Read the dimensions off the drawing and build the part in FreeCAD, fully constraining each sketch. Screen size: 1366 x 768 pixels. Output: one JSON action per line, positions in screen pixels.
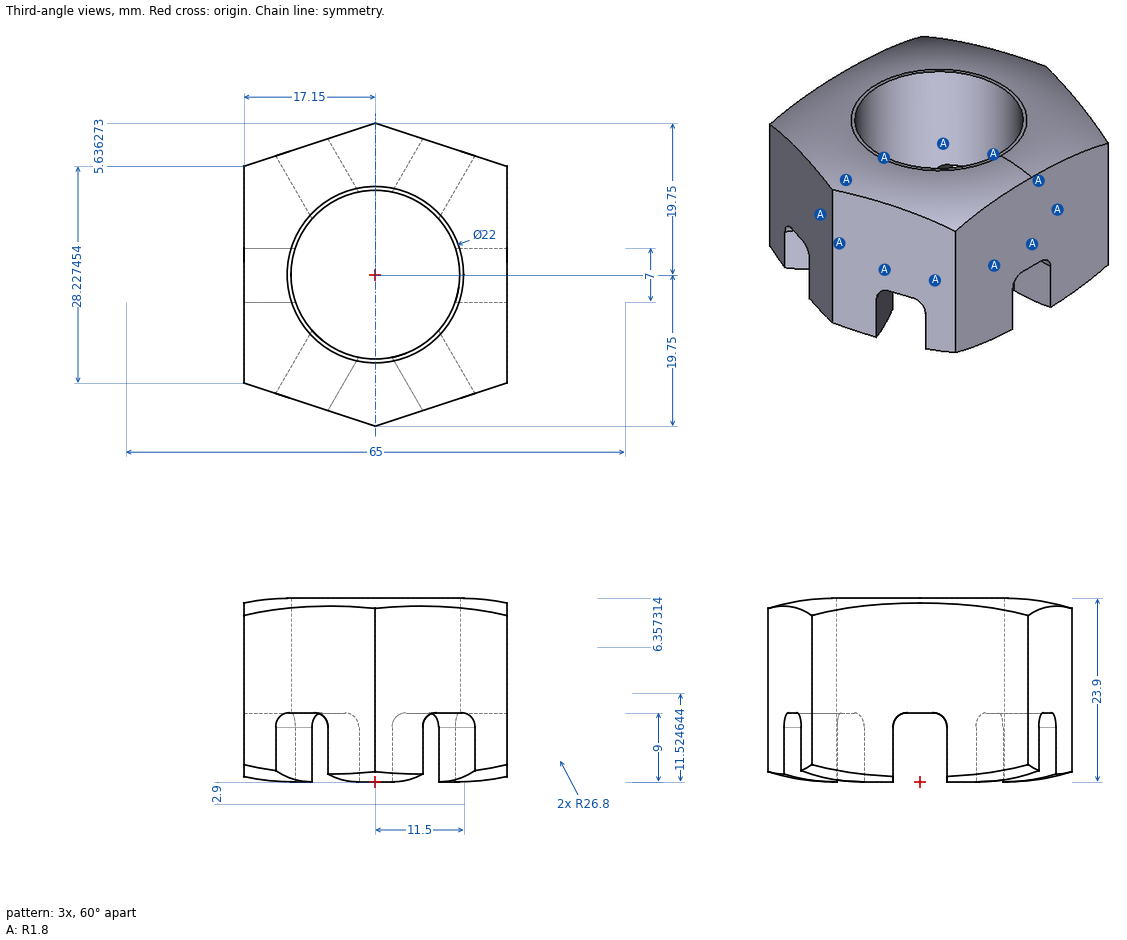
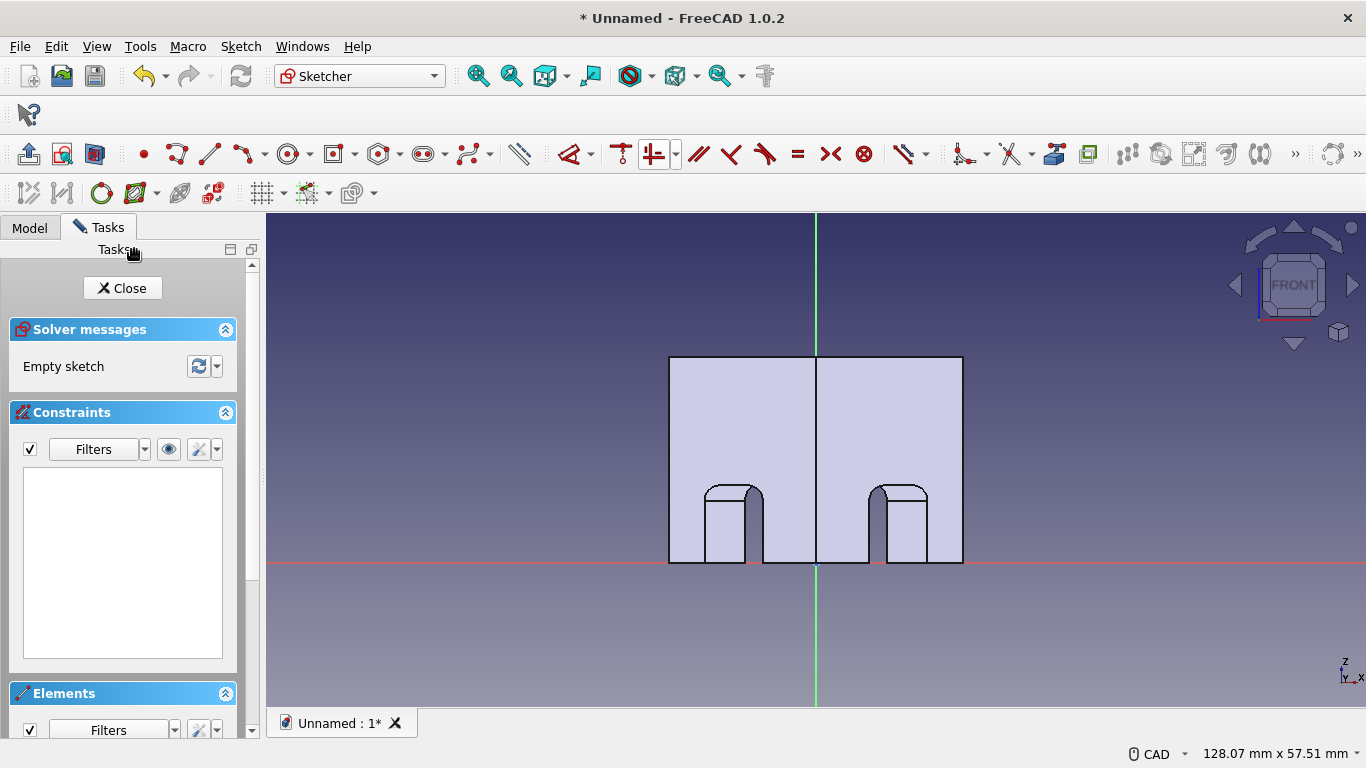
{"action": "left_click", "coordinate": [95, 154]}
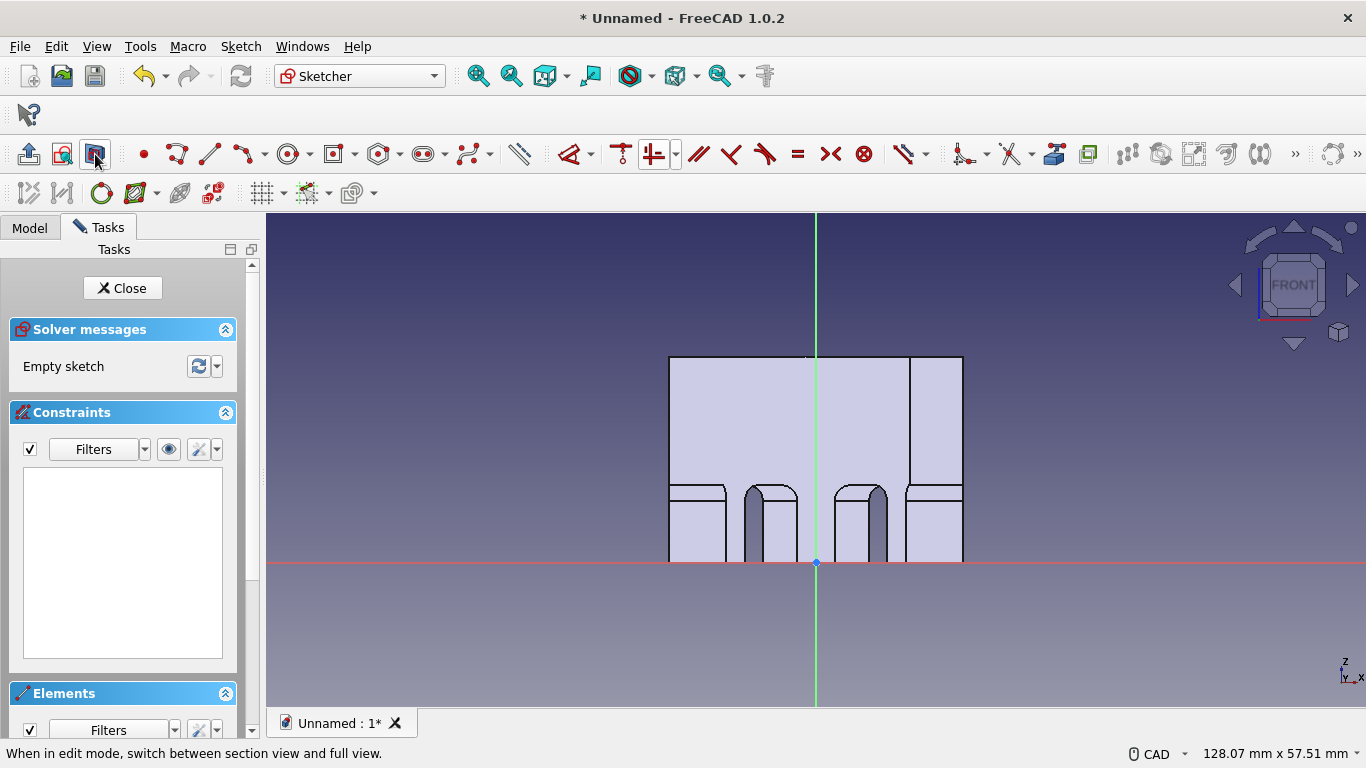
{"action": "scroll", "coordinate": [1201, 460], "scroll_direction": "up", "scroll_amount": 2}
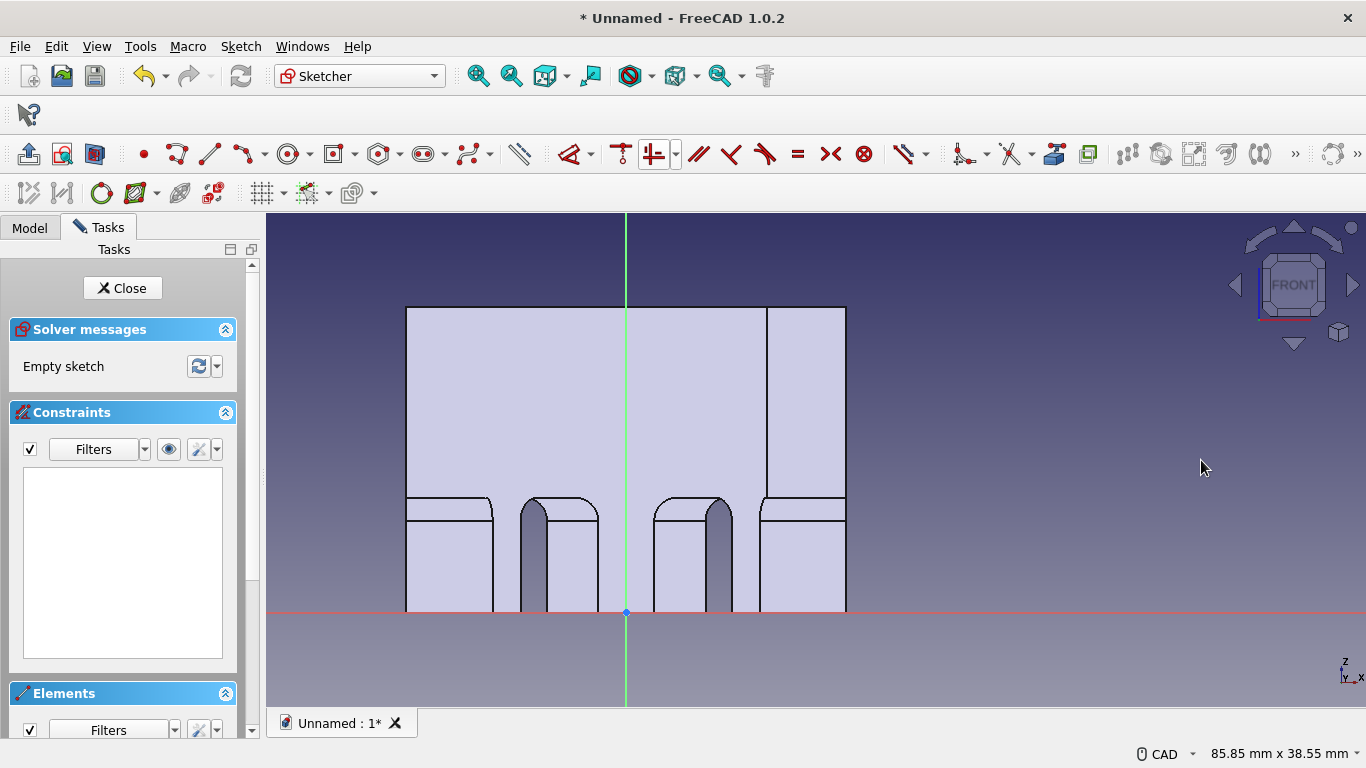
{"action": "left_click", "coordinate": [177, 154]}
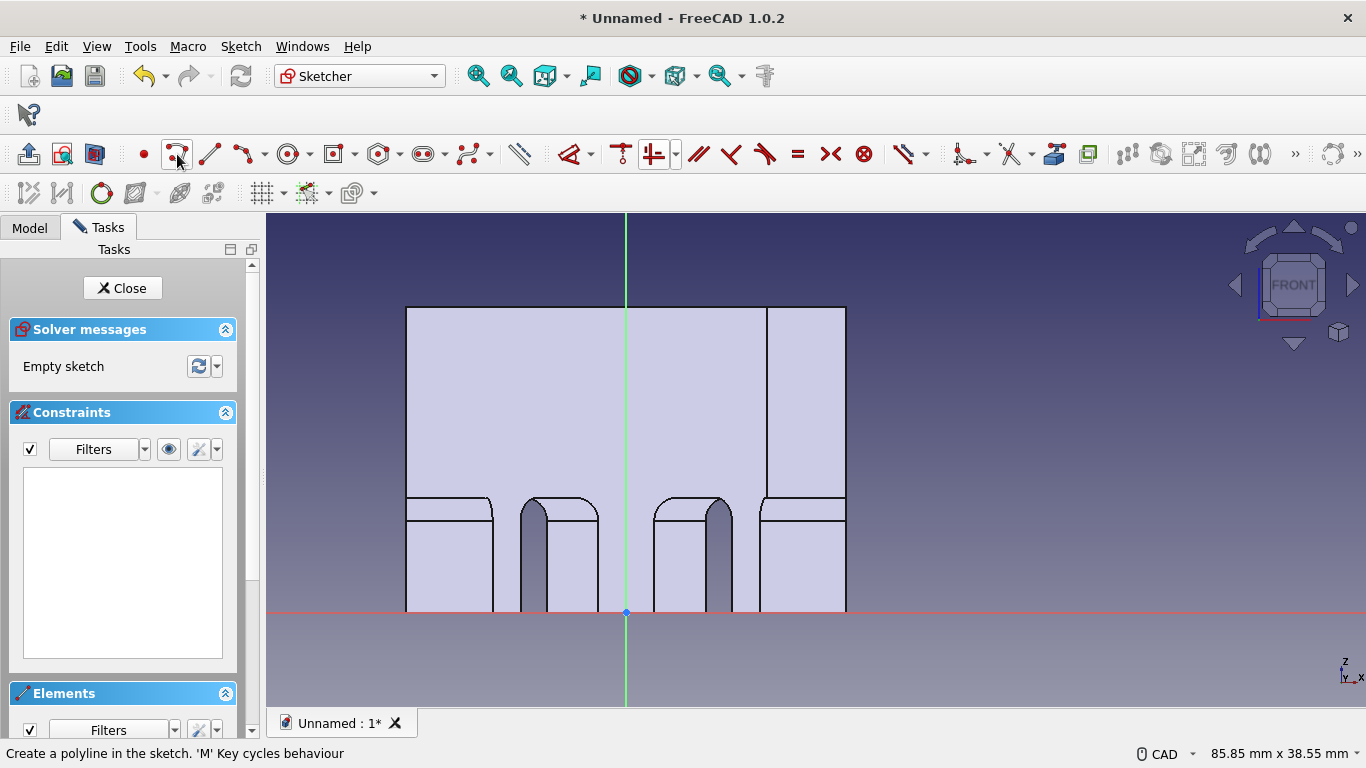
{"action": "left_click", "coordinate": [1056, 465]}
{"action": "left_click", "coordinate": [1056, 613]}
{"action": "left_click", "coordinate": [774, 604]}
{"action": "right_click", "coordinate": [774, 604]}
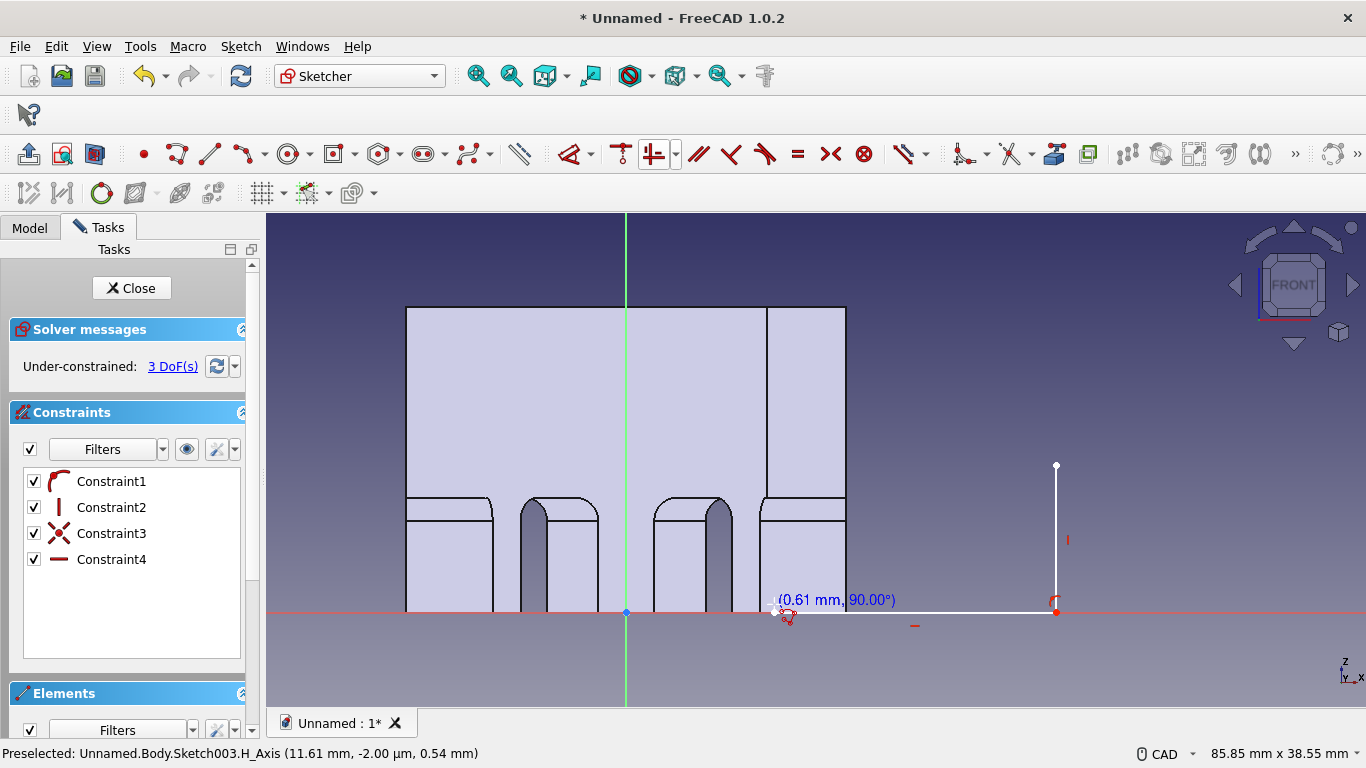
{"action": "left_click", "coordinate": [242, 154]}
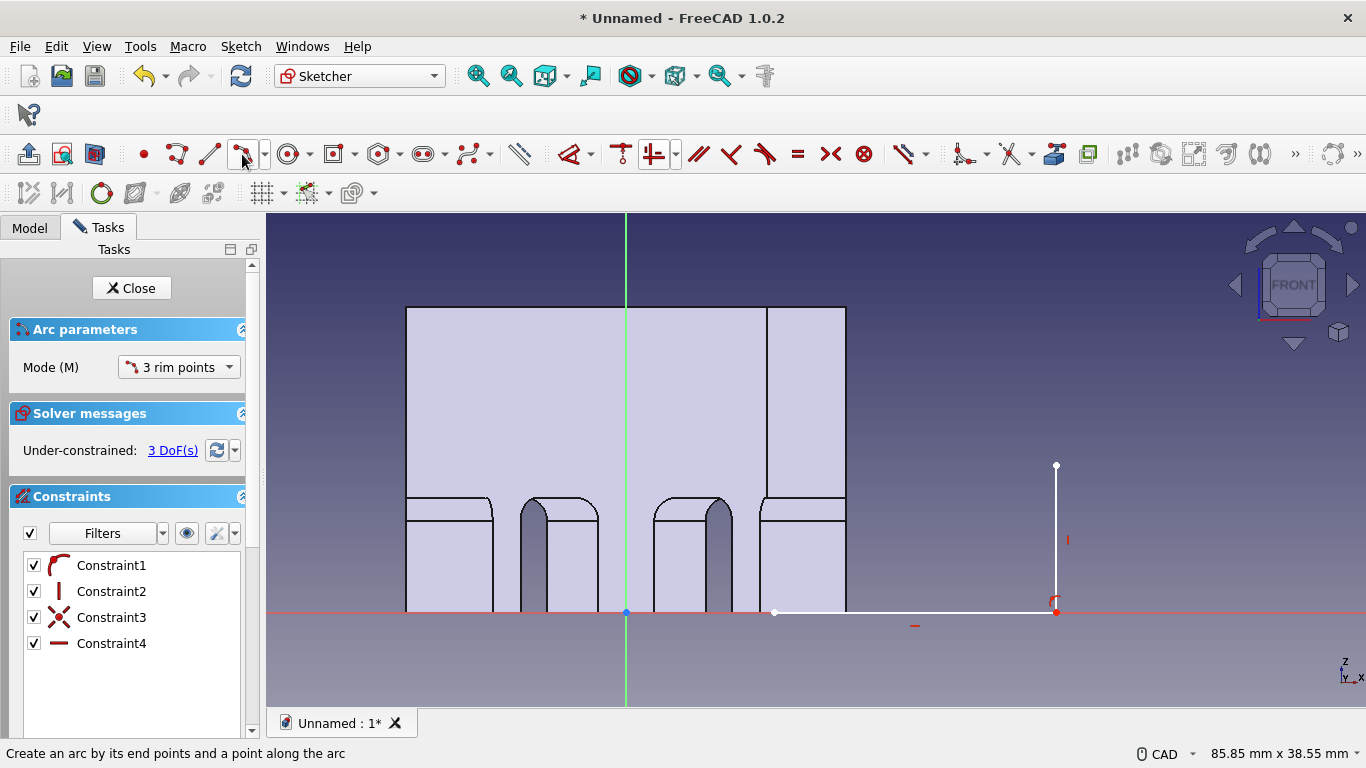
{"action": "left_click", "coordinate": [774, 613]}
{"action": "left_click", "coordinate": [1056, 466]}
{"action": "left_click", "coordinate": [933, 574]}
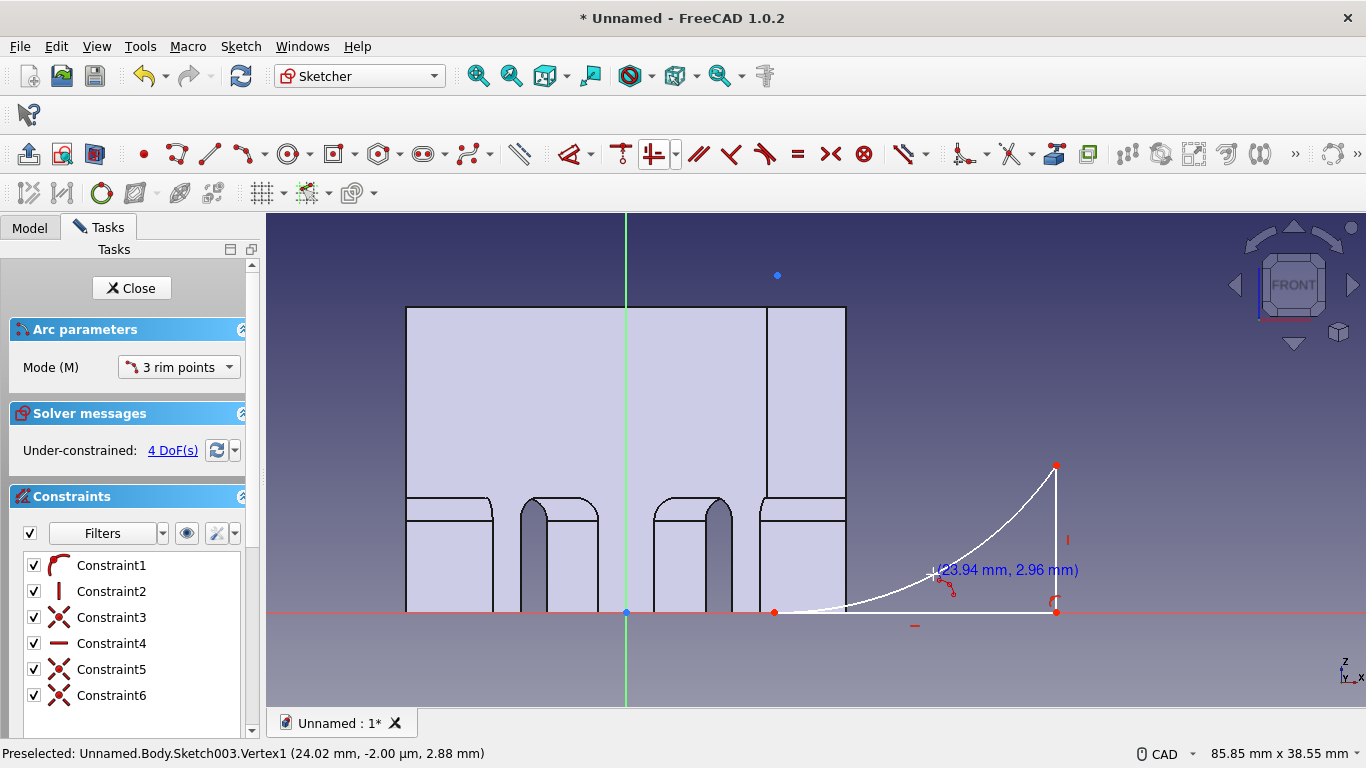
{"action": "left_click", "coordinate": [177, 154]}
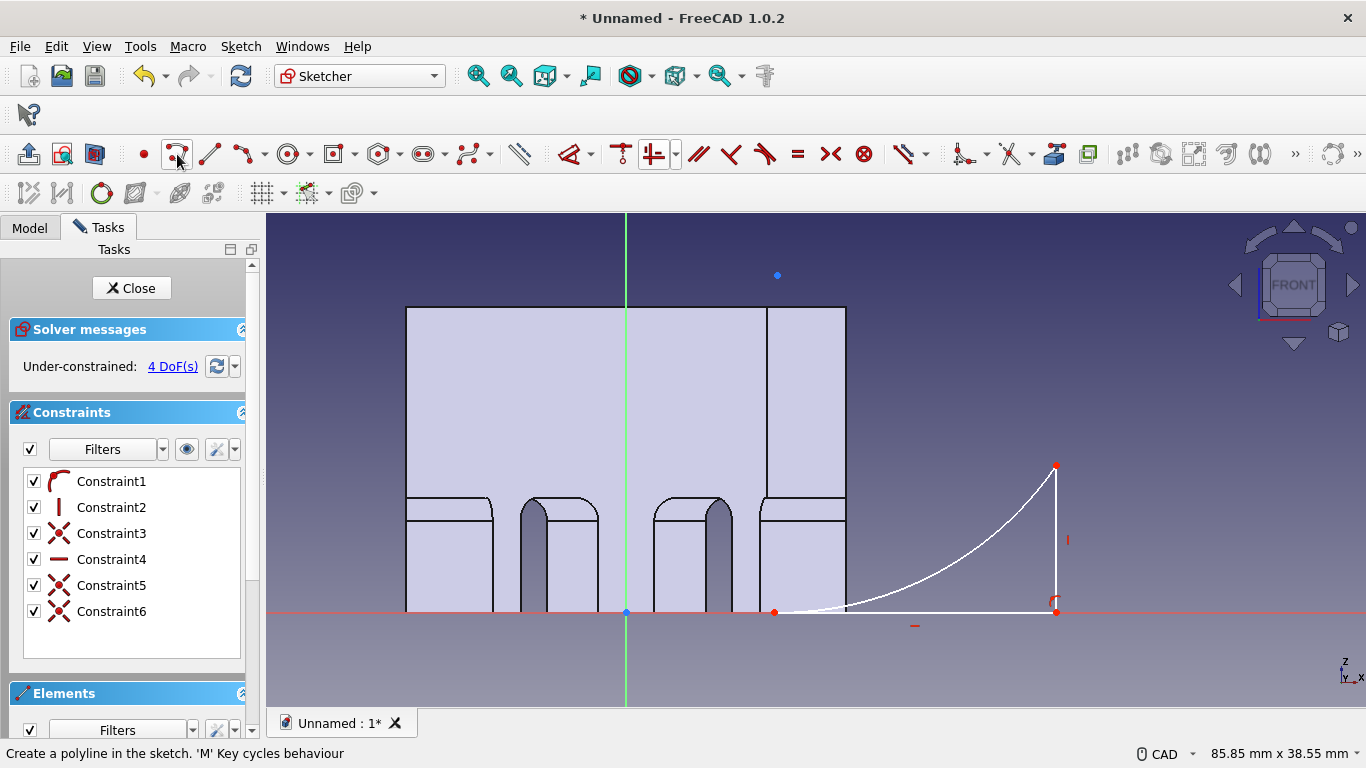
{"action": "left_click", "coordinate": [774, 307]}
{"action": "left_click", "coordinate": [996, 307]}
{"action": "left_click", "coordinate": [996, 388]}
{"action": "right_click", "coordinate": [996, 388]}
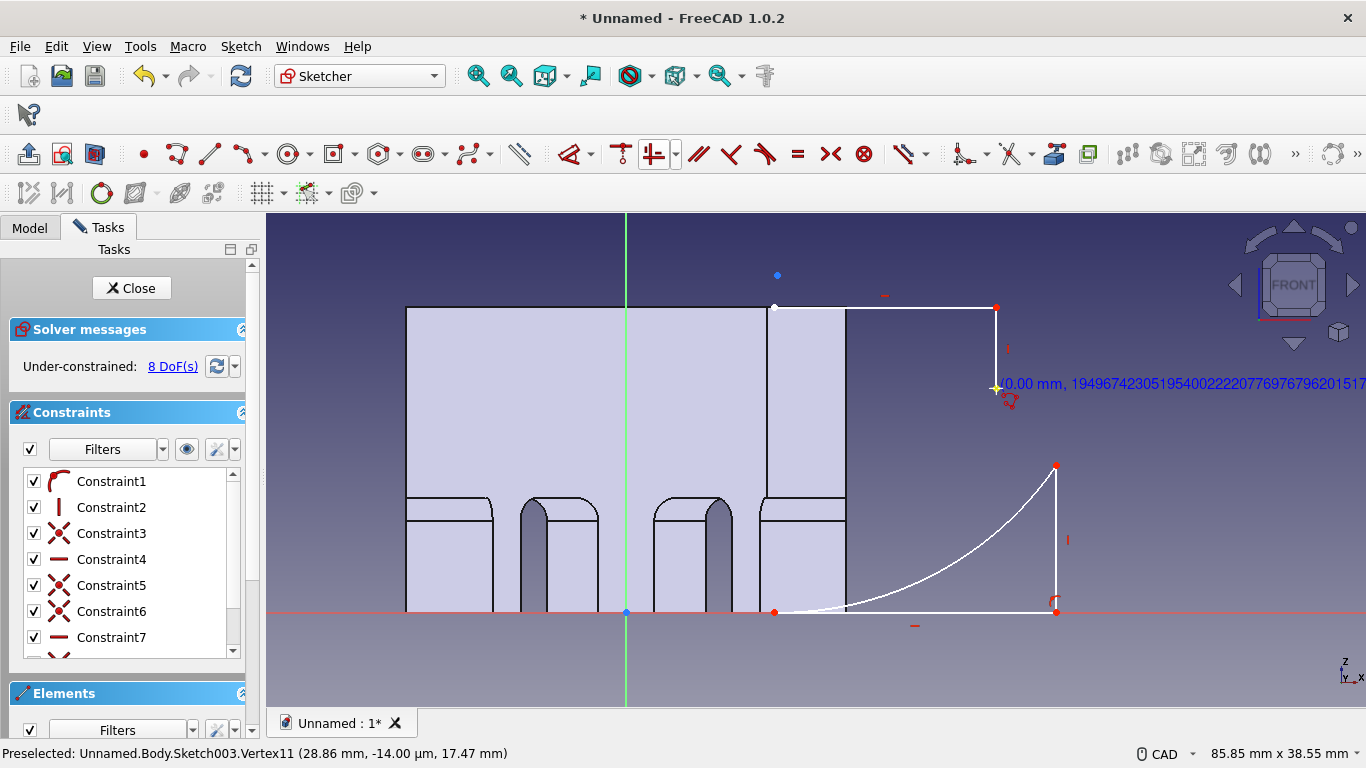
{"action": "left_click", "coordinate": [242, 154]}